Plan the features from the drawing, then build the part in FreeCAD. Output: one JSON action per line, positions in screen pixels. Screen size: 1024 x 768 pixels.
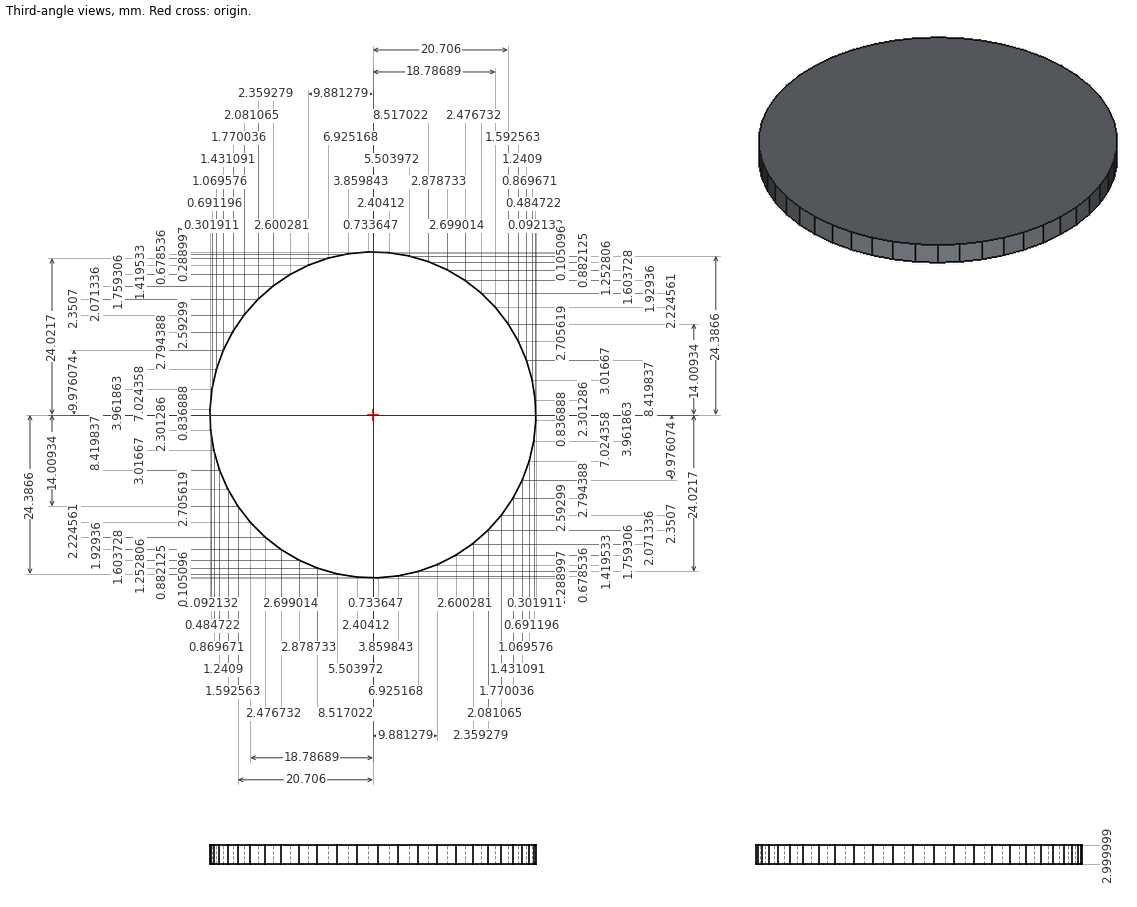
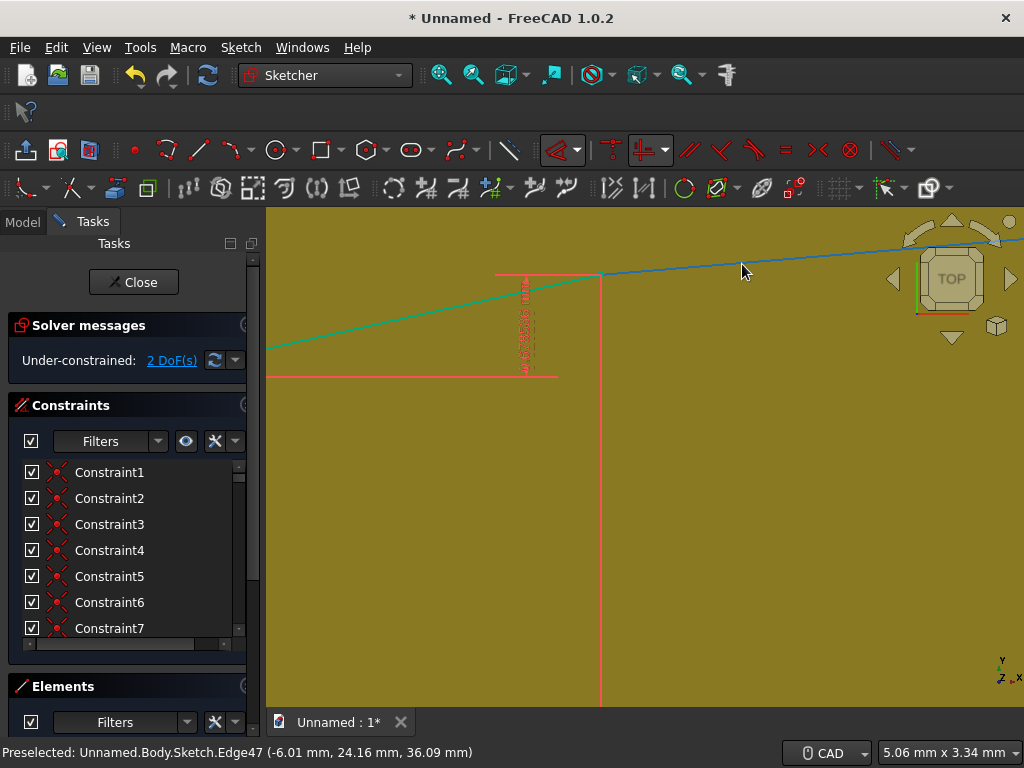
{"action": "left_click", "coordinate": [741, 263]}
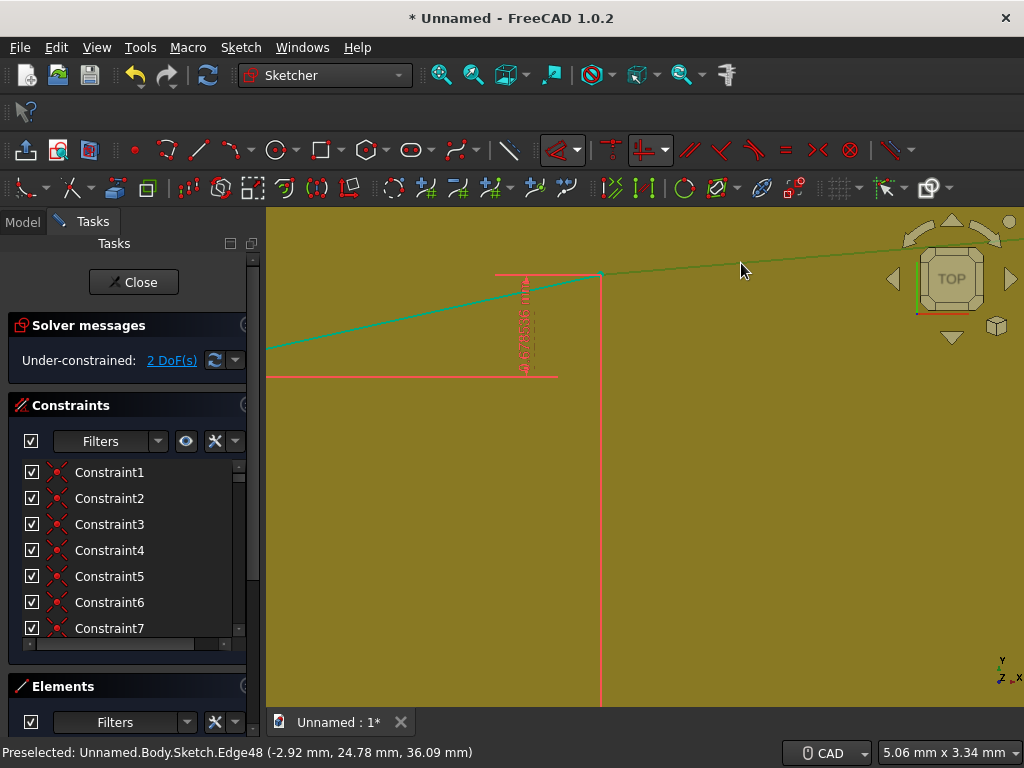
{"action": "key", "text": "i"}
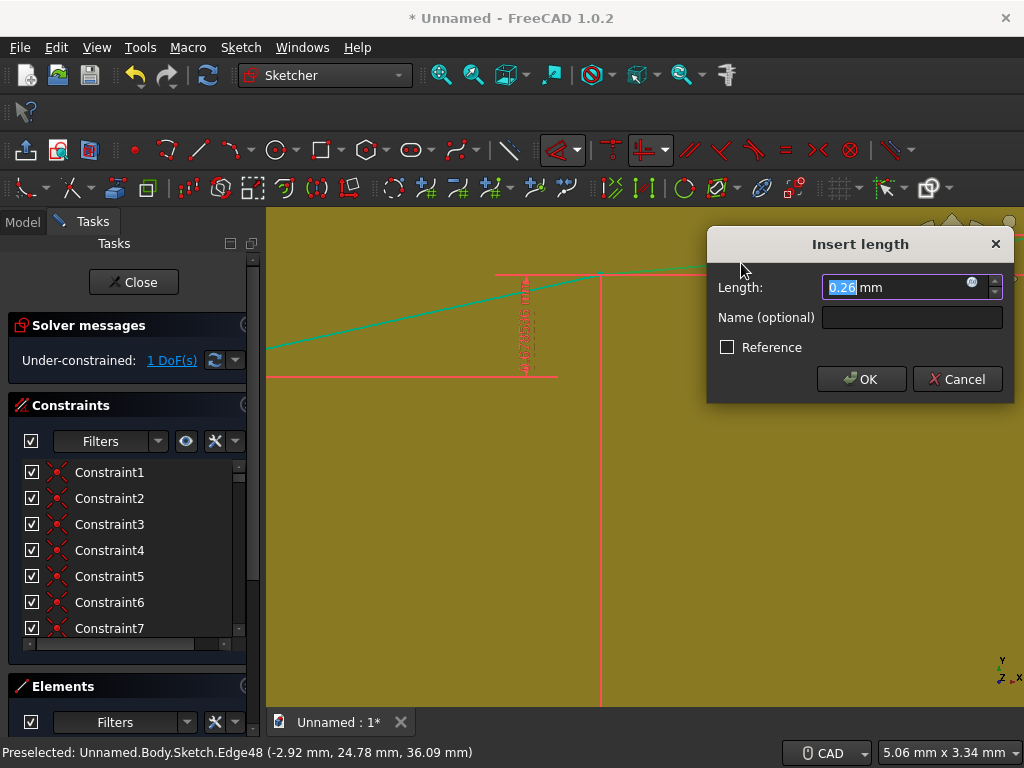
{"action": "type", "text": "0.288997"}
{"action": "key", "text": "Return"}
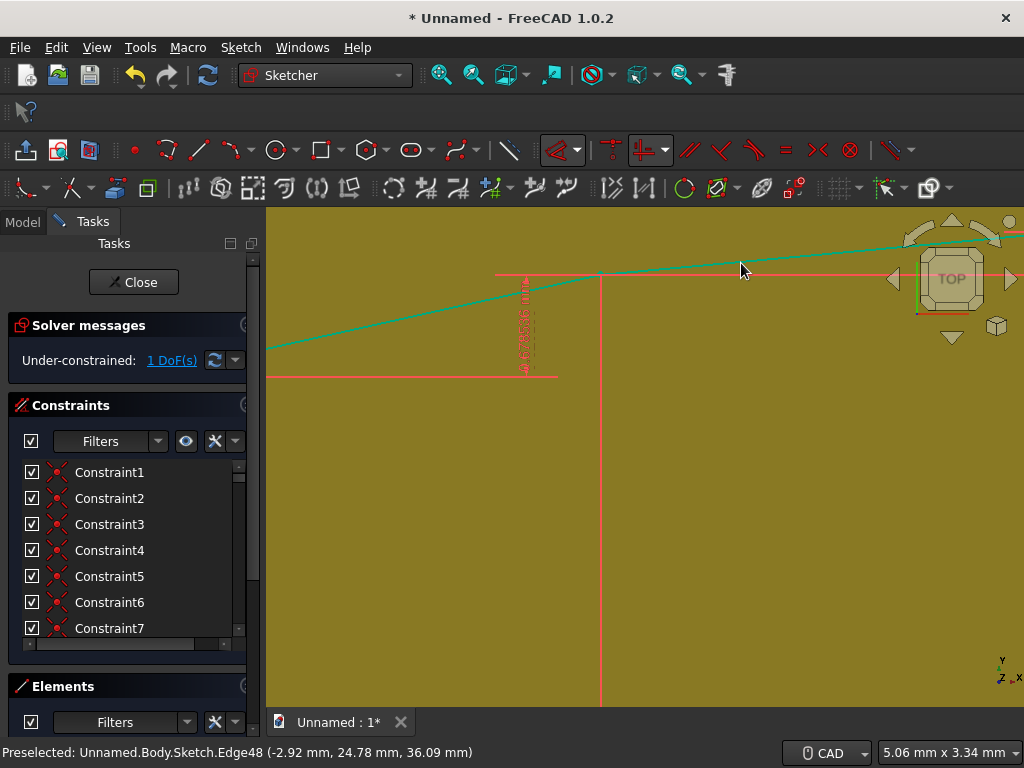
{"action": "scroll", "coordinate": [545, 273], "scroll_direction": "down", "scroll_amount": 15}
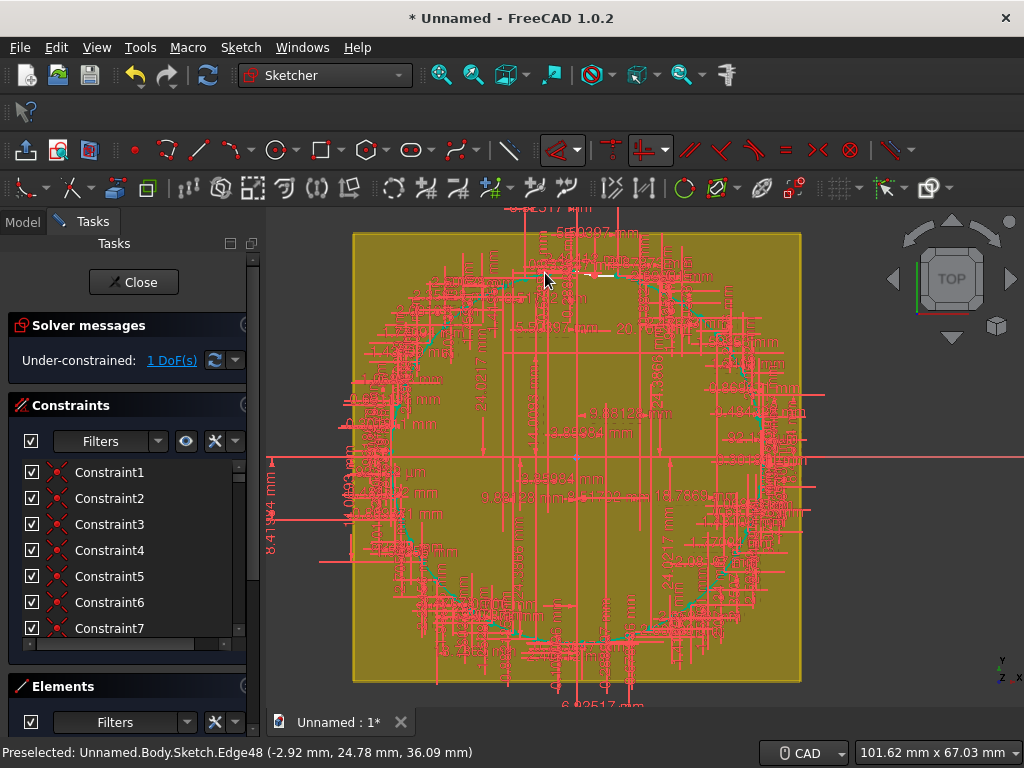
{"action": "scroll", "coordinate": [578, 272], "scroll_direction": "up", "scroll_amount": 20}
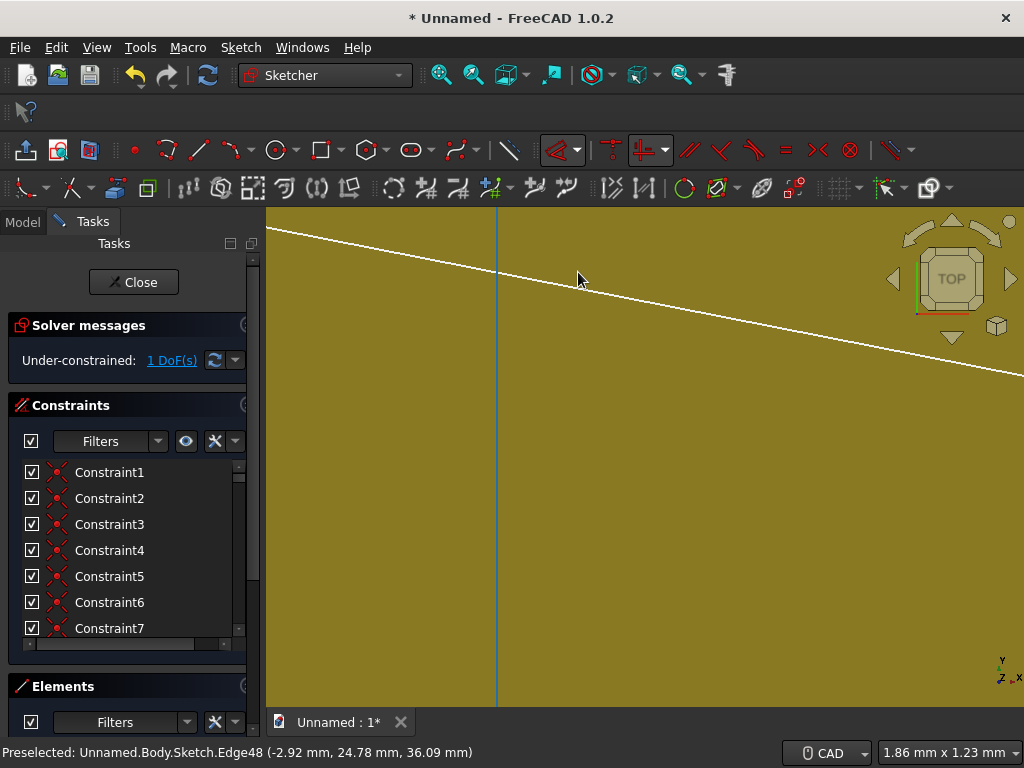
{"action": "left_click", "coordinate": [581, 289]}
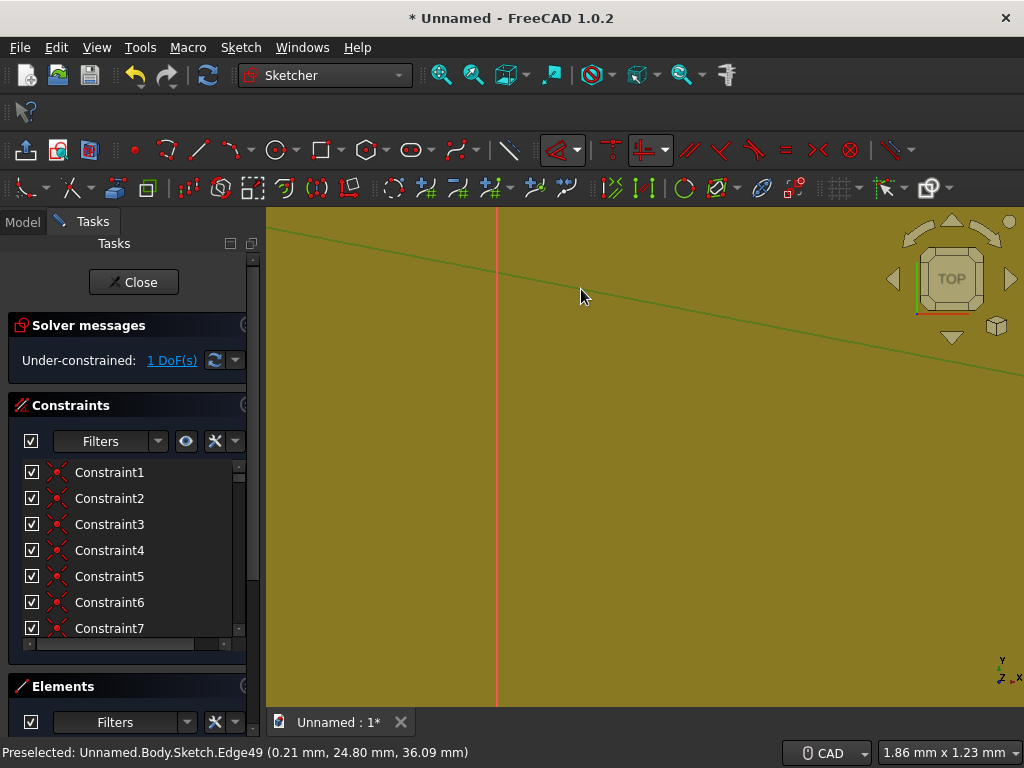
{"action": "key", "text": "i"}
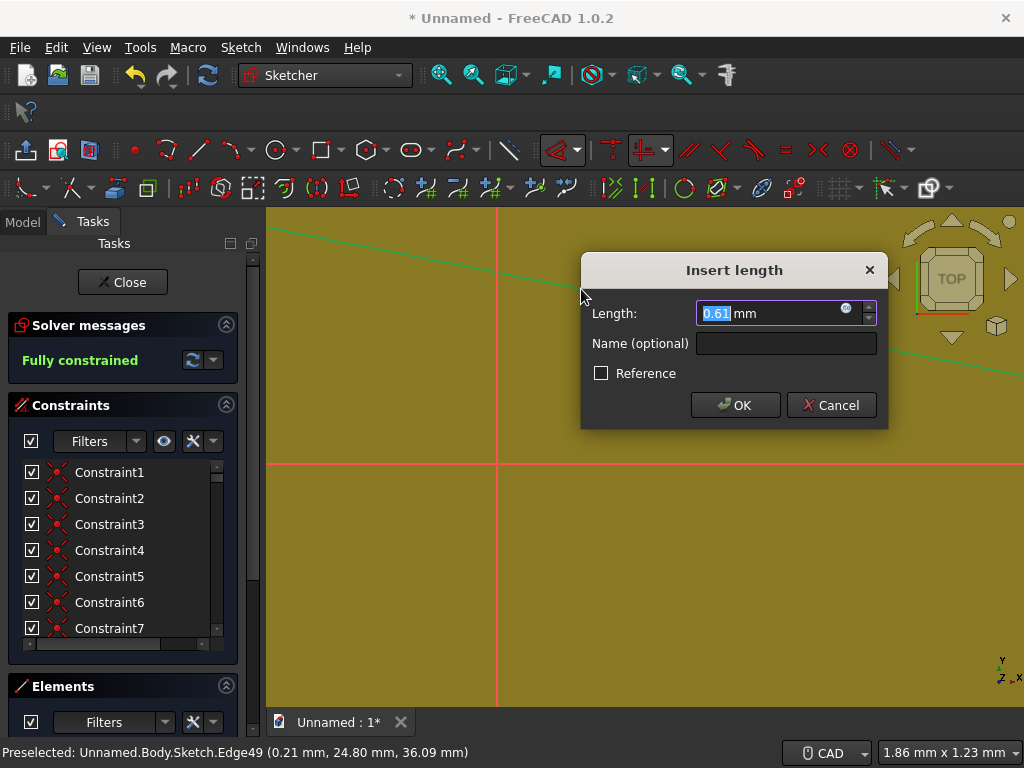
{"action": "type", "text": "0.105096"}
{"action": "key", "text": "Return"}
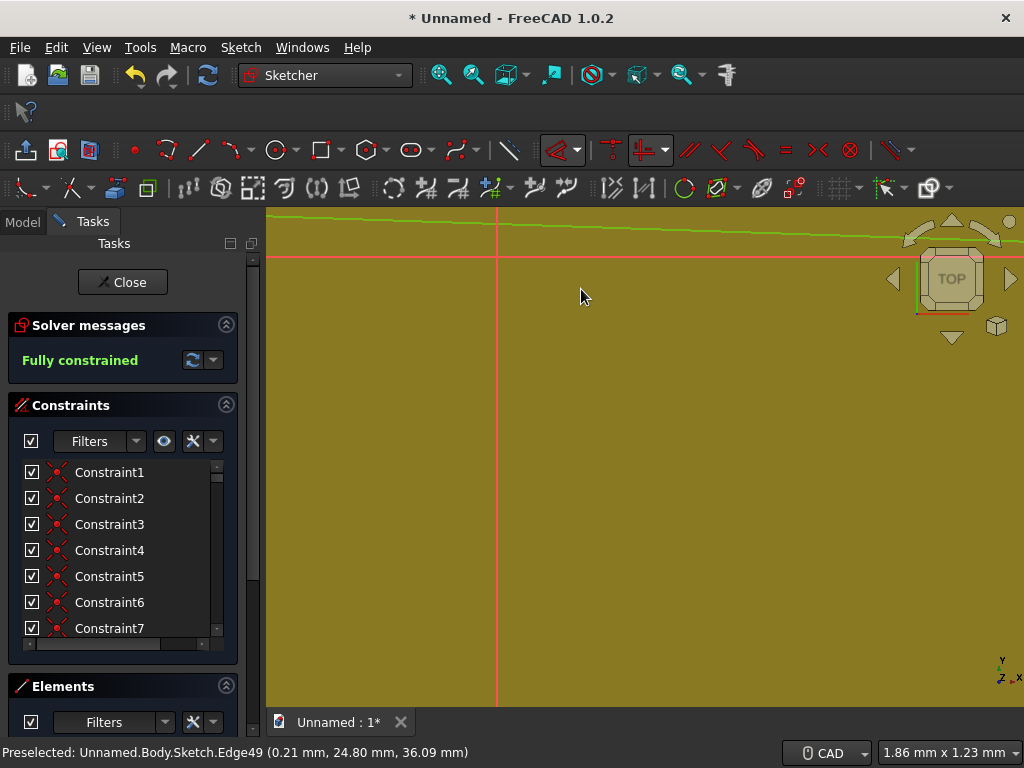
{"action": "left_click", "coordinate": [123, 282]}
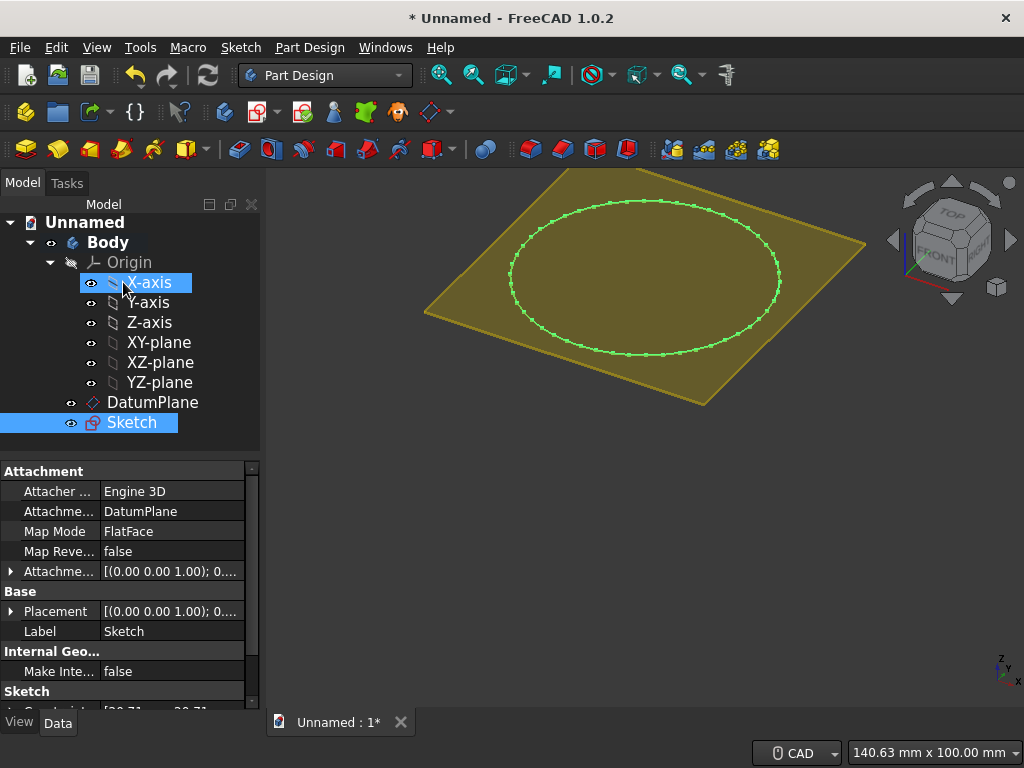
{"action": "left_click", "coordinate": [26, 150]}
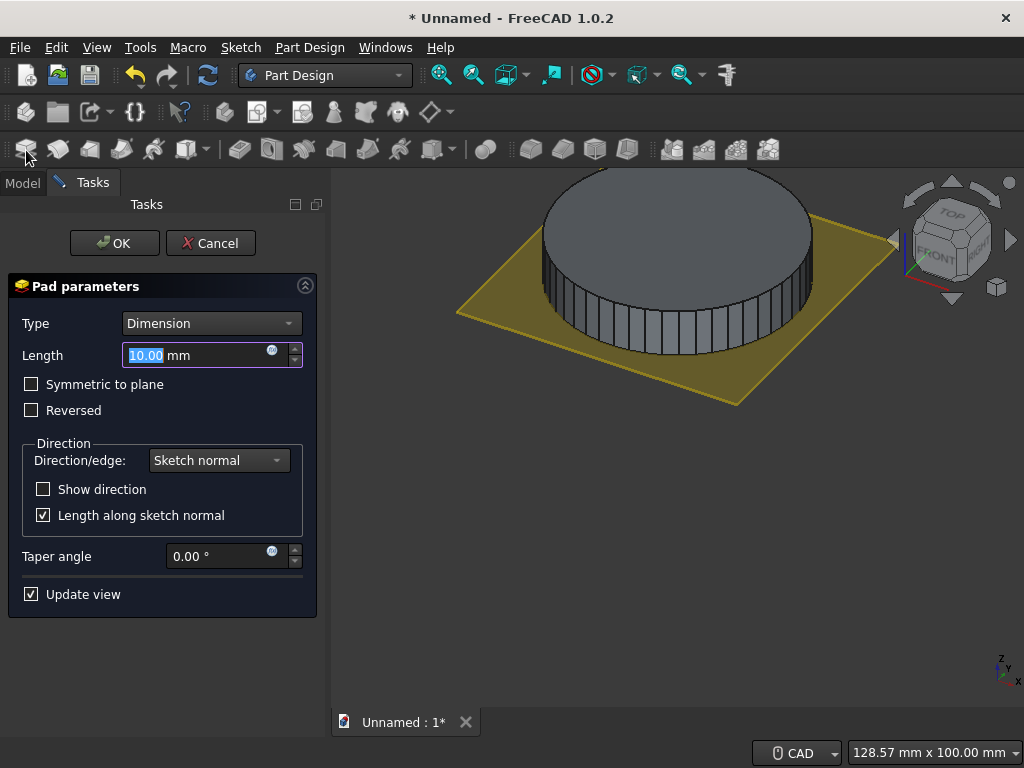
{"action": "type", "text": "2.999999"}
{"action": "key", "text": "Tab"}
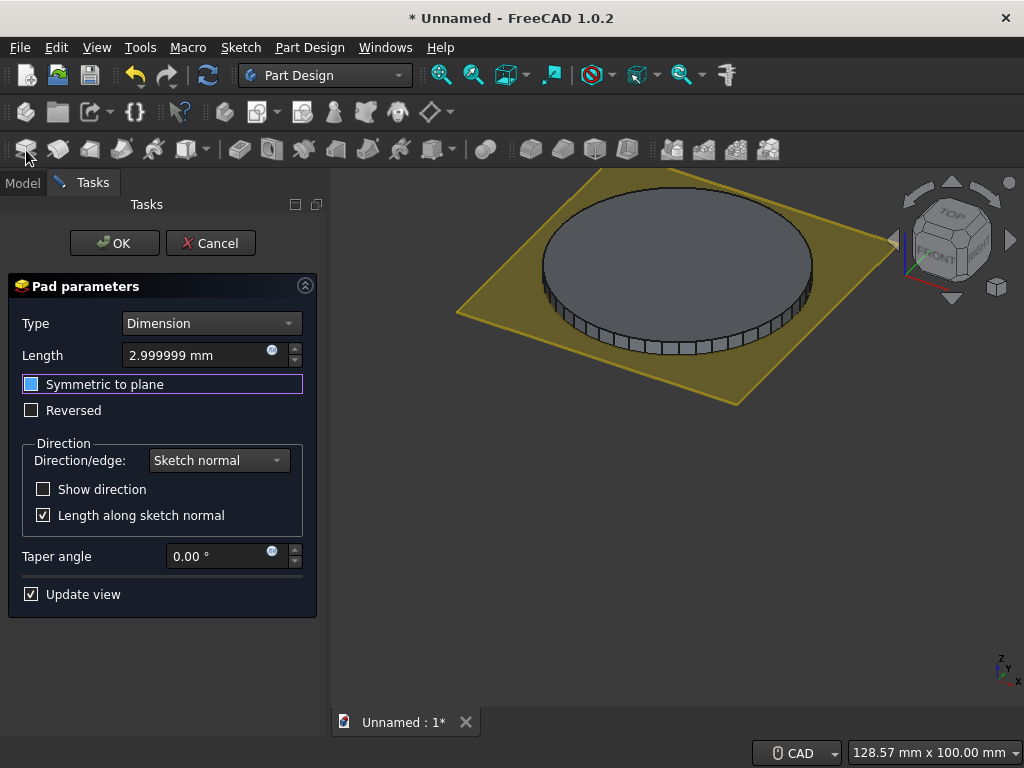
{"action": "left_click", "coordinate": [115, 243]}